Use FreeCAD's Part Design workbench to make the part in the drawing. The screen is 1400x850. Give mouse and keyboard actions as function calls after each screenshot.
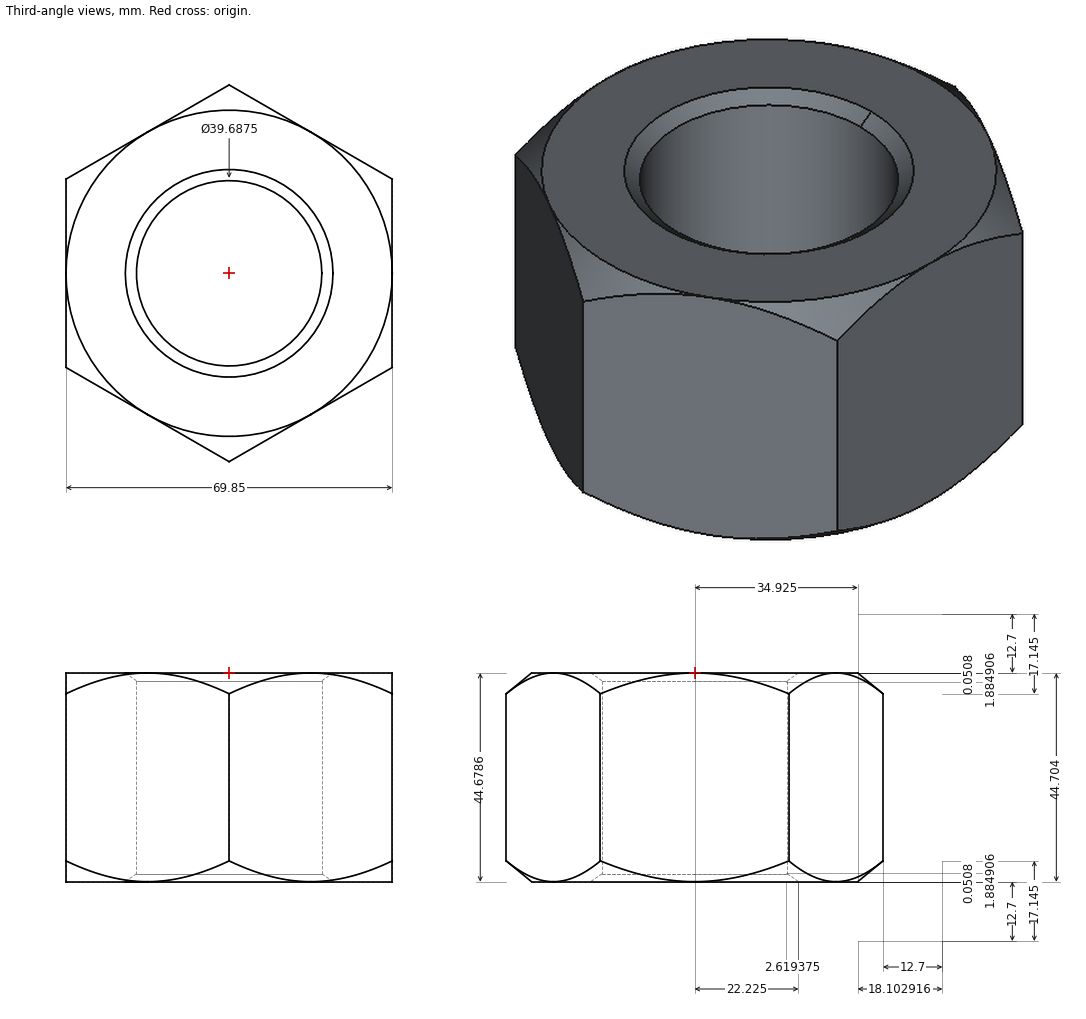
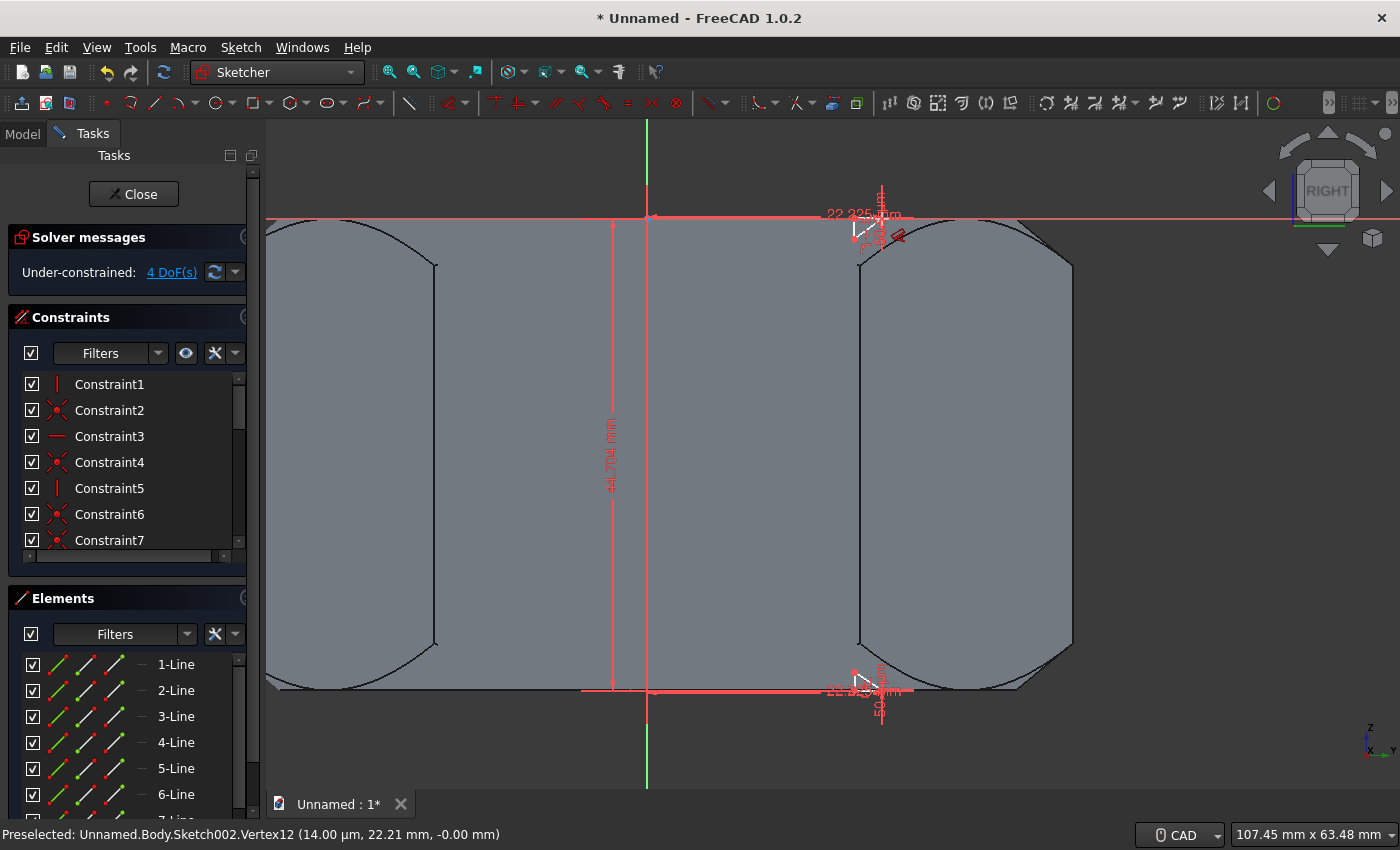
scroll(855, 678, up, 6)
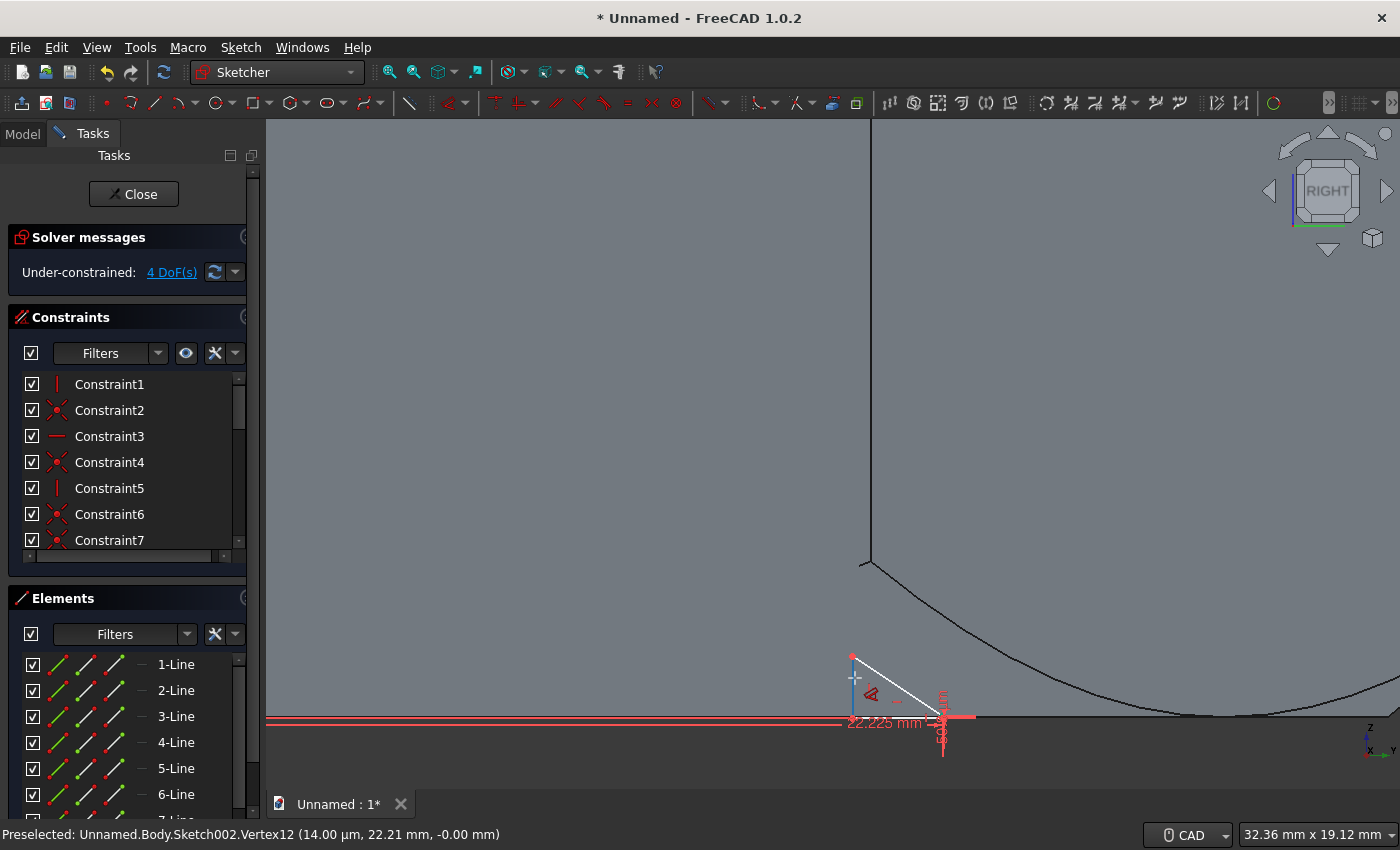
click(853, 675)
click(819, 687)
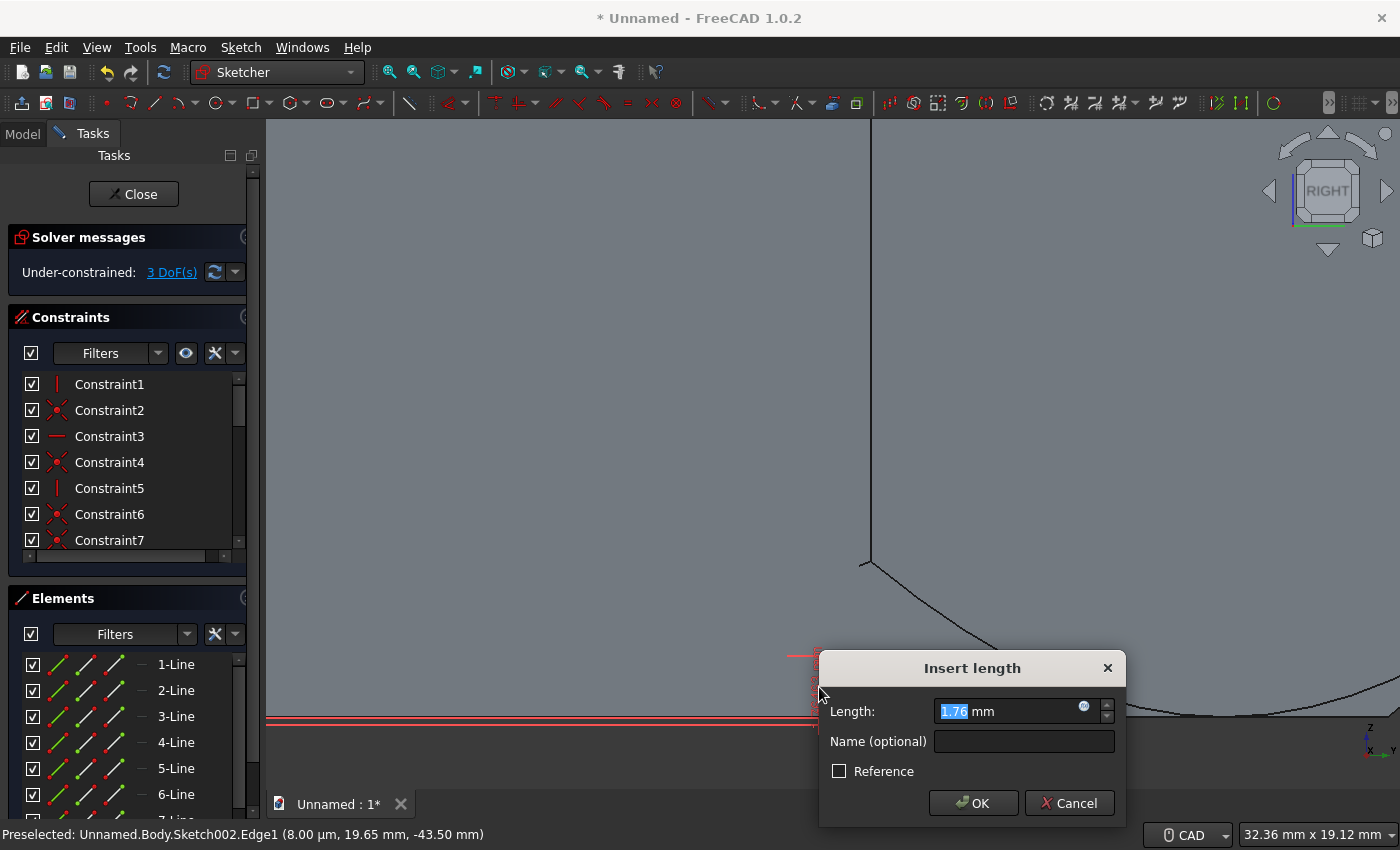
text(1.884906)
key(Return)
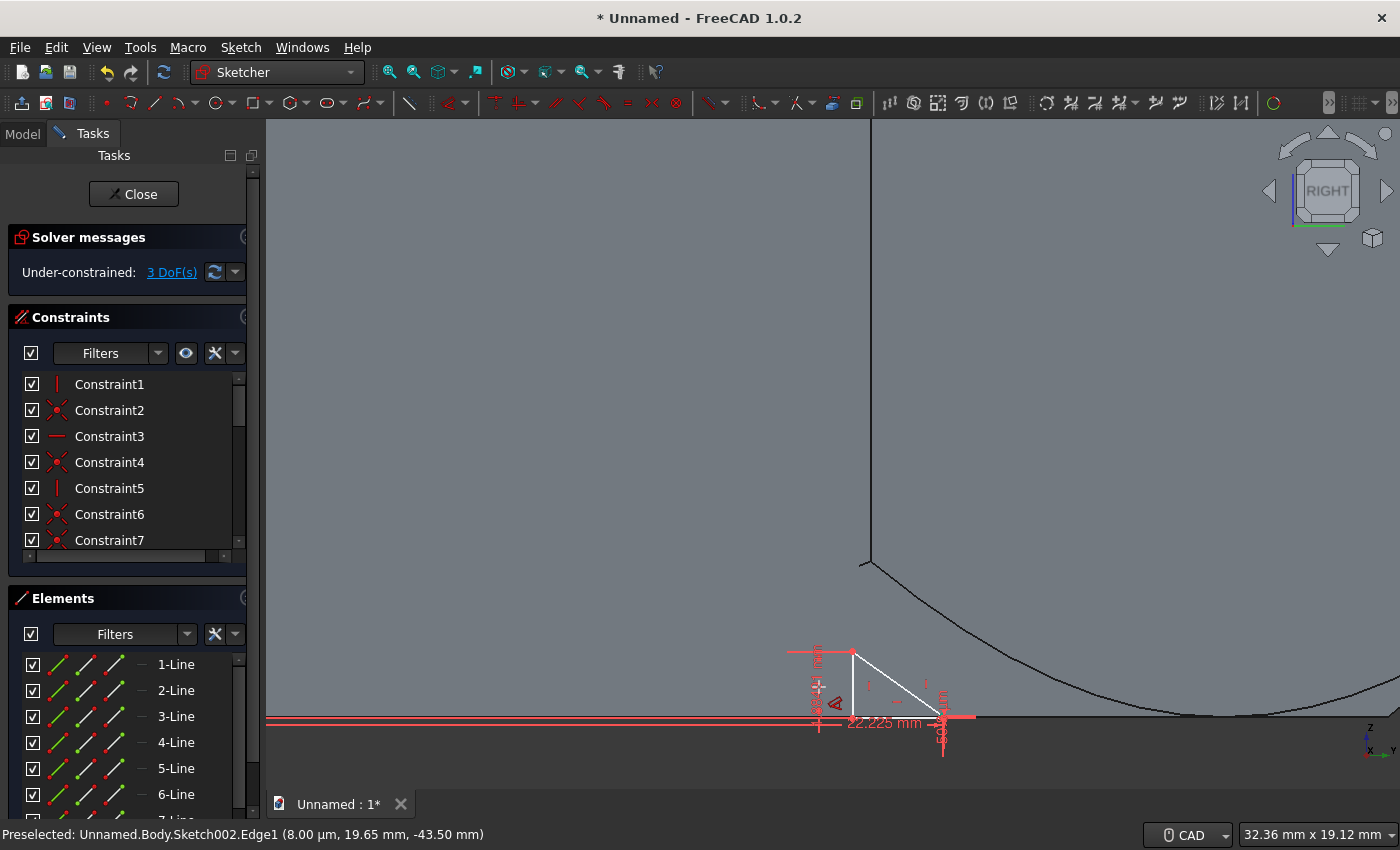
click(880, 718)
click(898, 752)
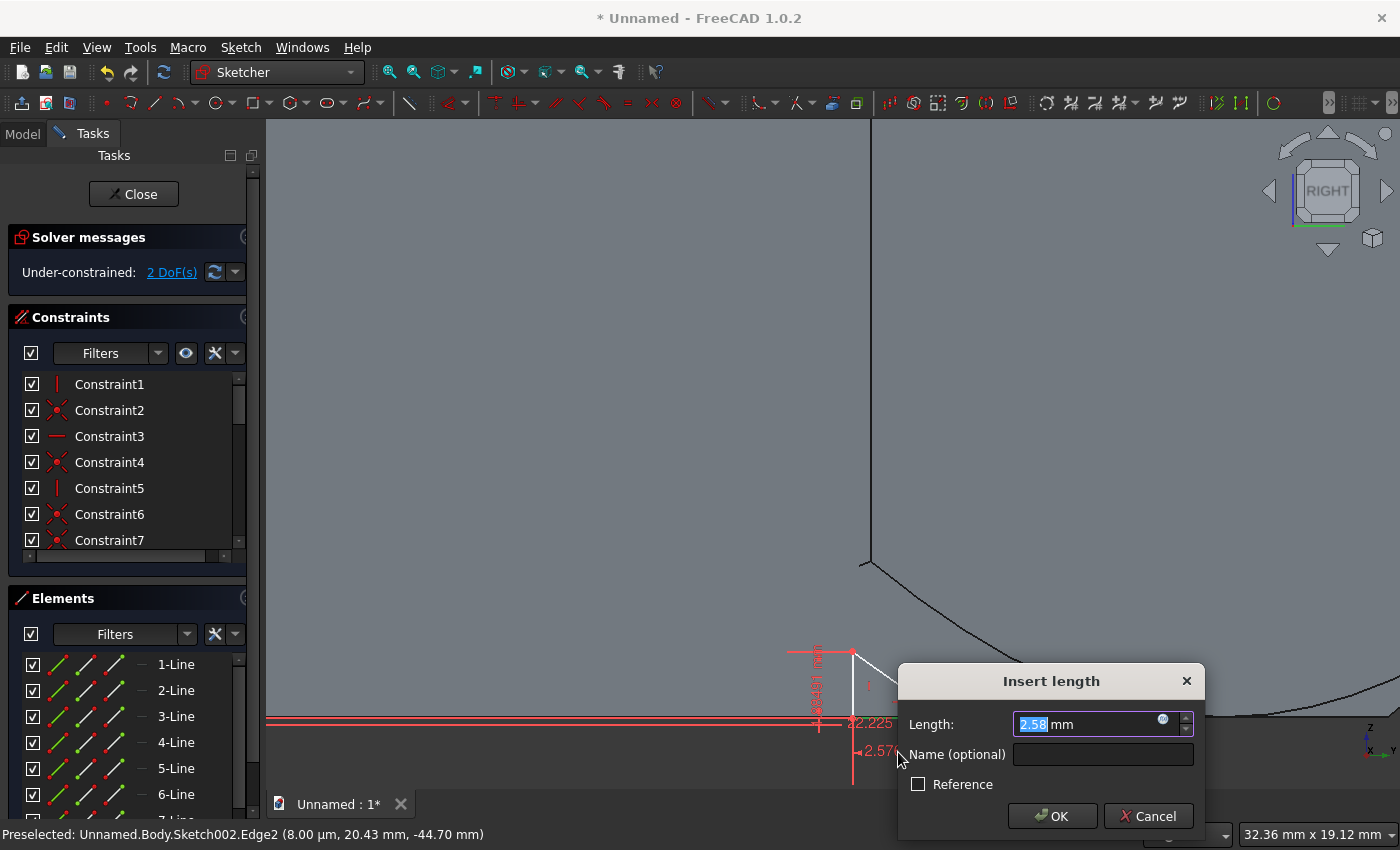
text(2.619375)
key(Return)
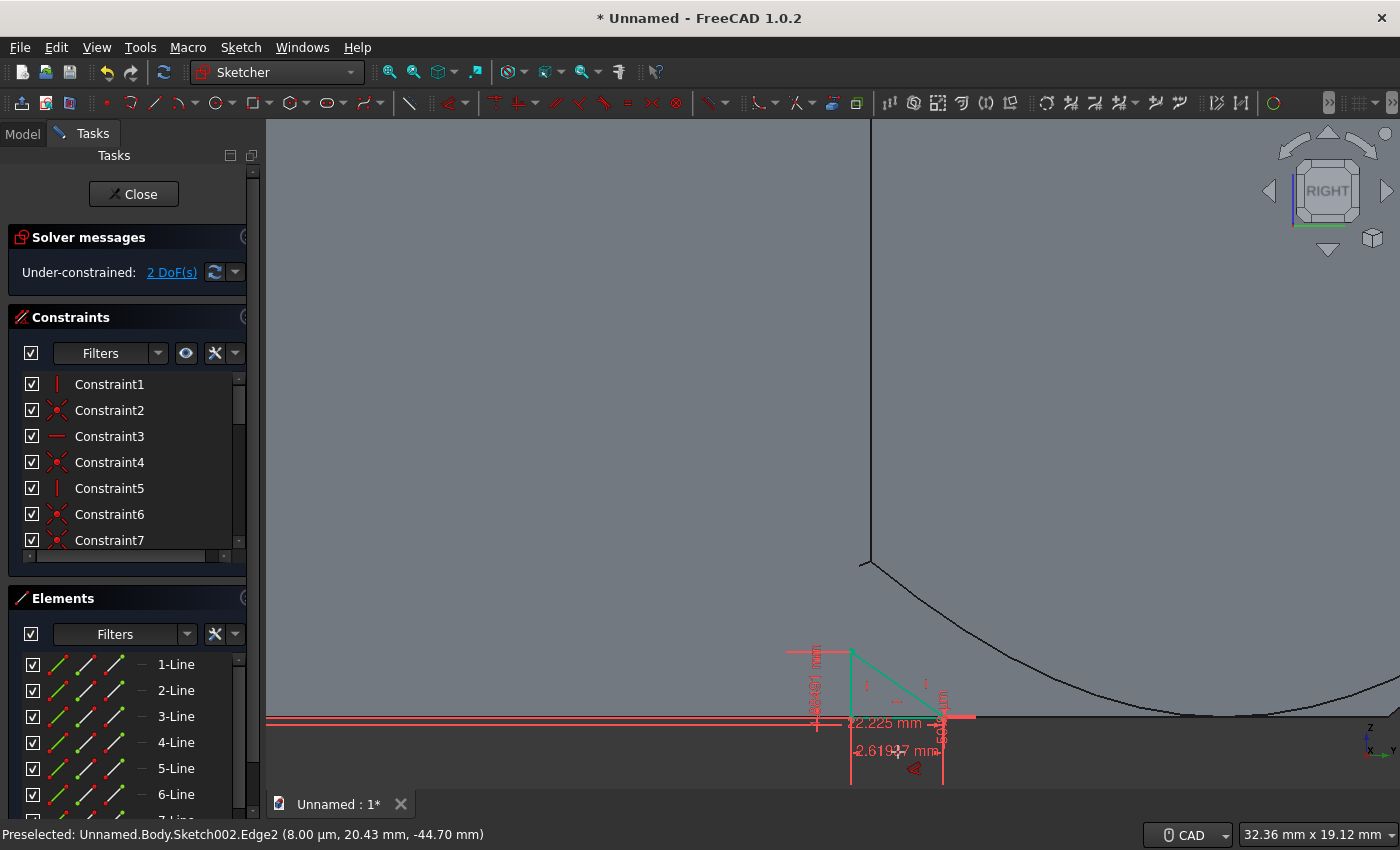
scroll(855, 678, down, 6)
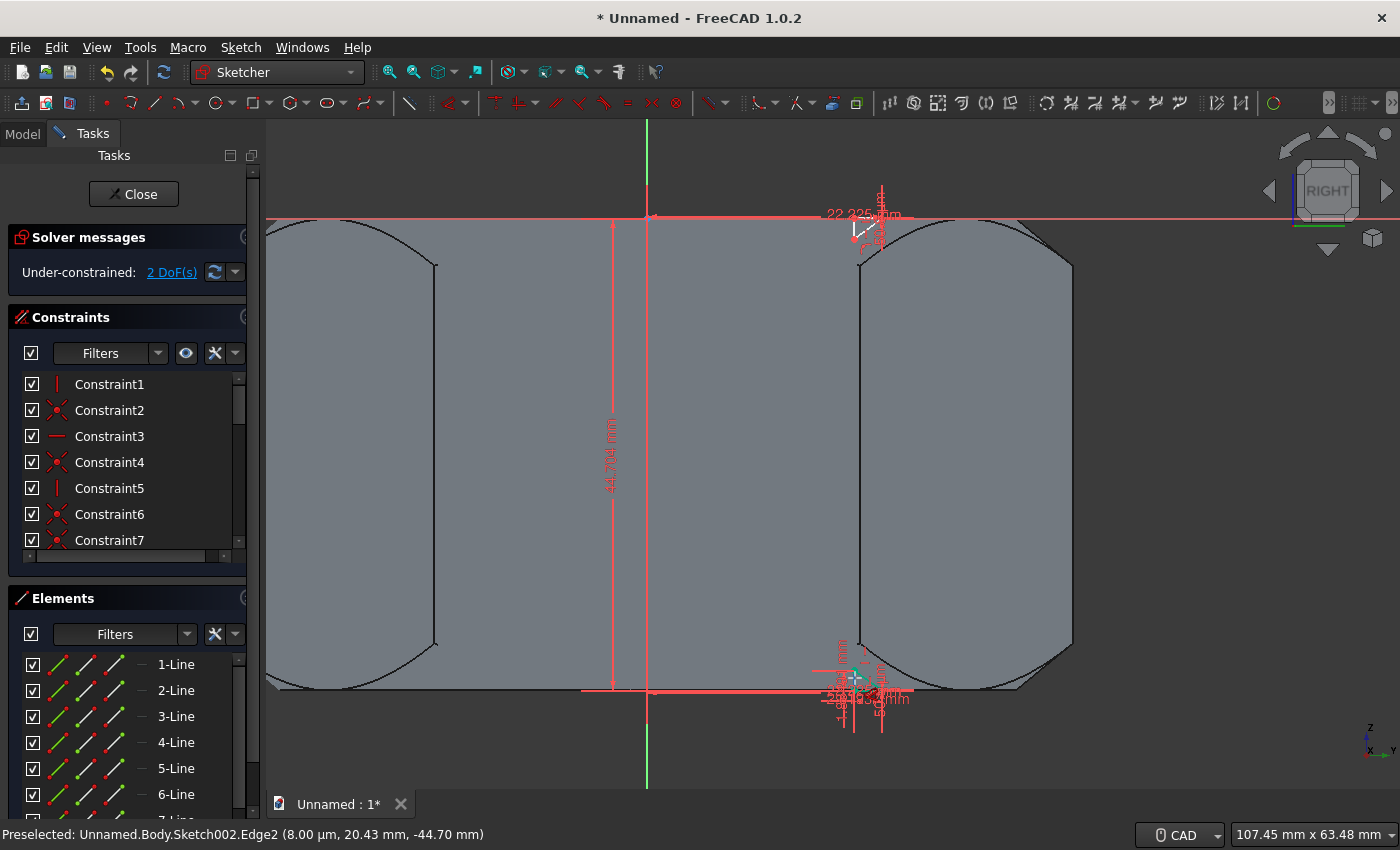
scroll(854, 225, up, 5)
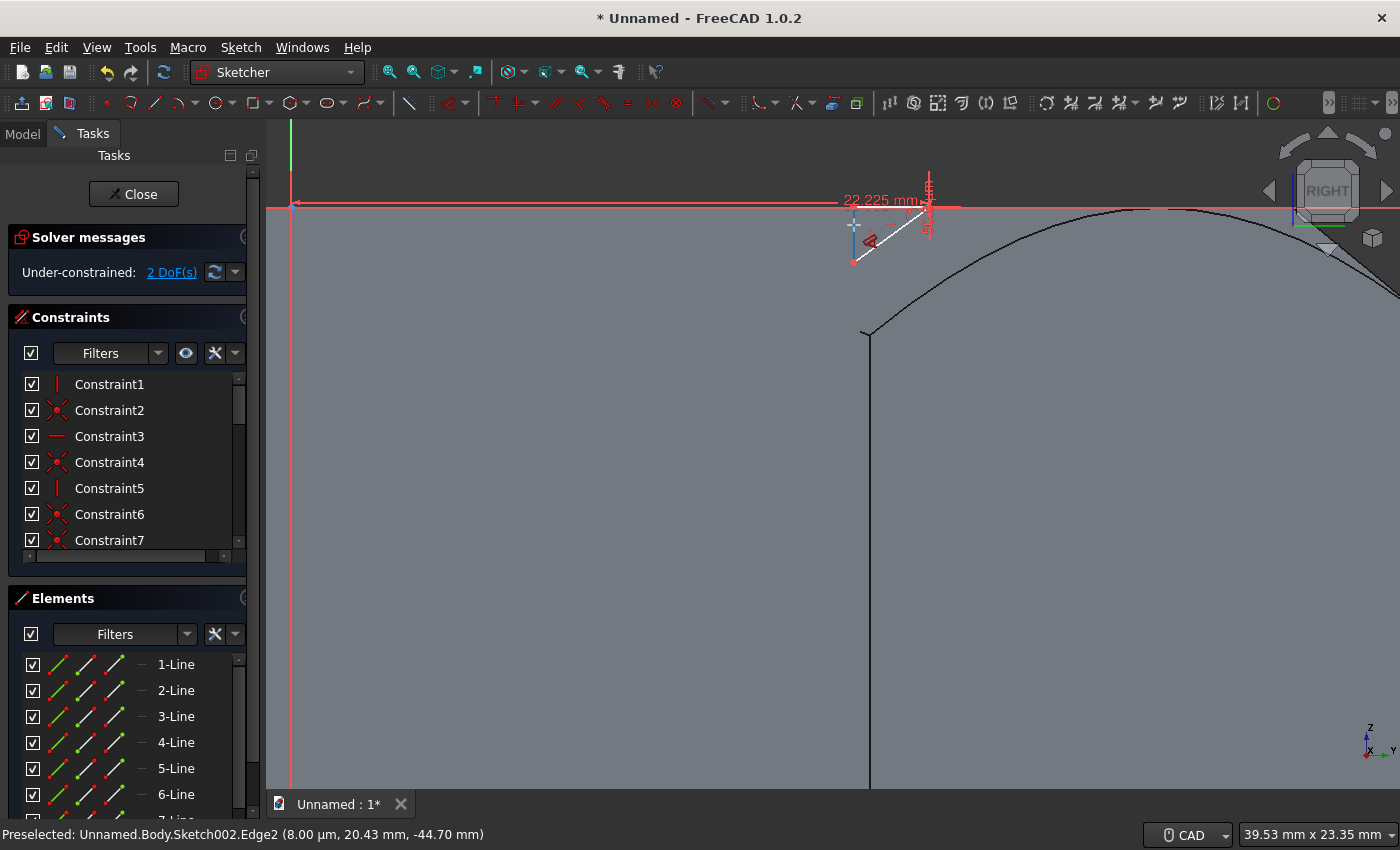
click(854, 223)
click(888, 254)